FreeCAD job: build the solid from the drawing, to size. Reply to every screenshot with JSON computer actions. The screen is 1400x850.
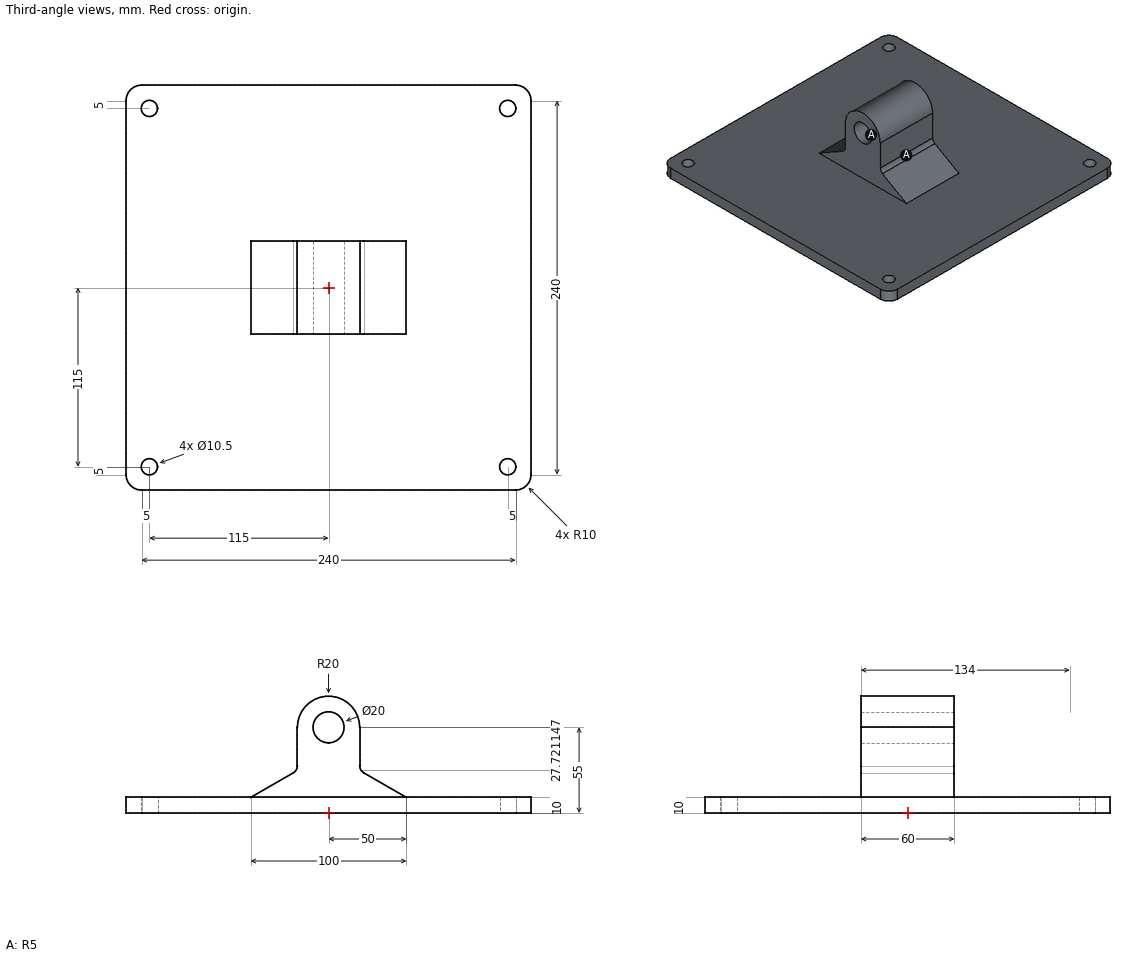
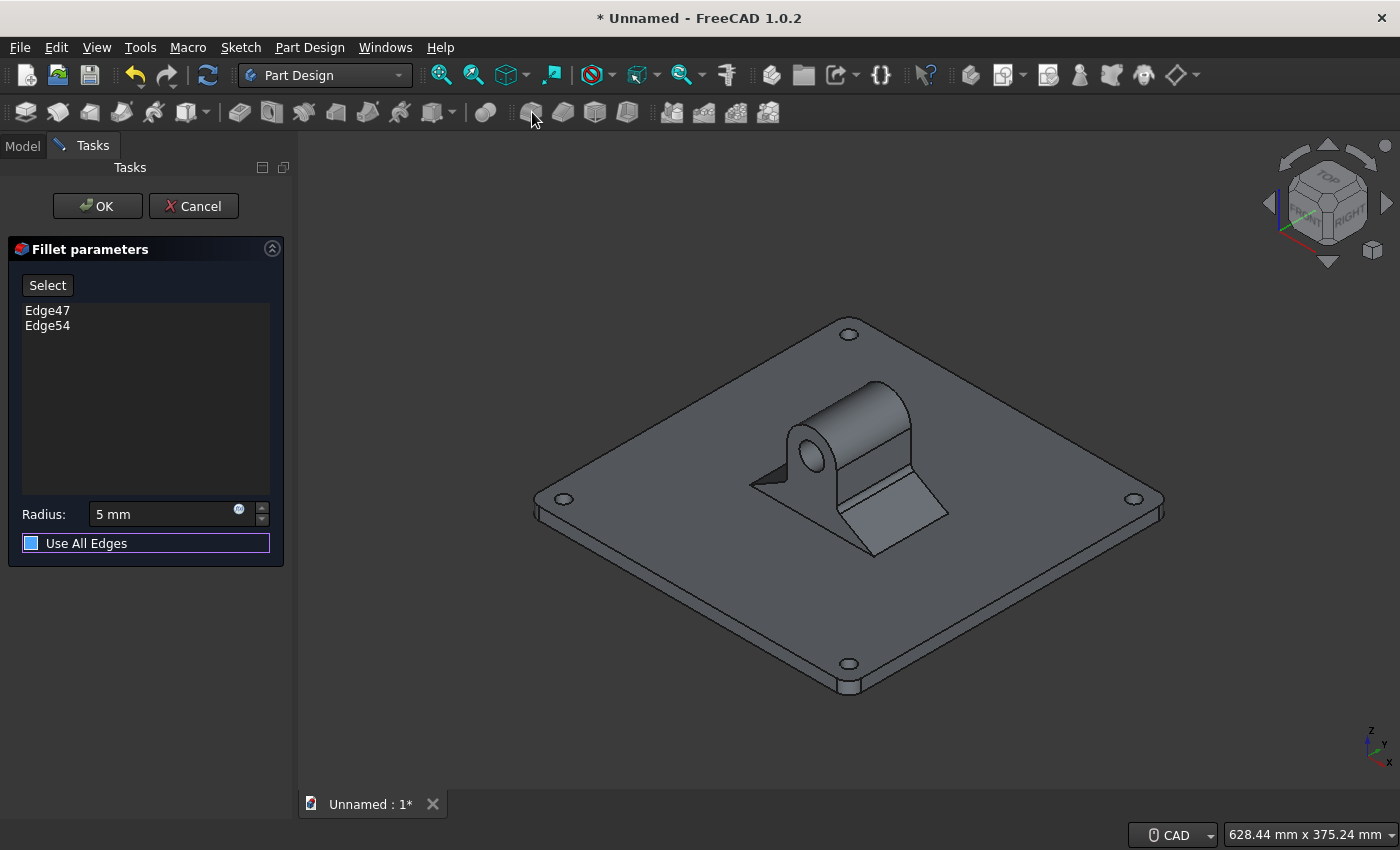
{"action": "left_click", "coordinate": [98, 206]}